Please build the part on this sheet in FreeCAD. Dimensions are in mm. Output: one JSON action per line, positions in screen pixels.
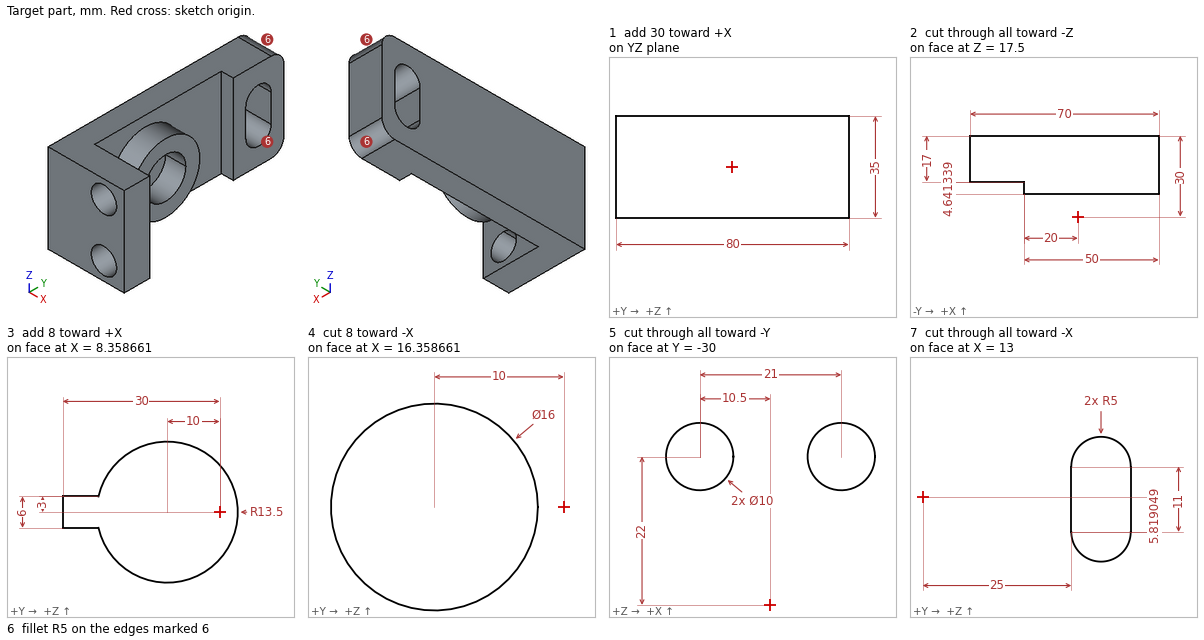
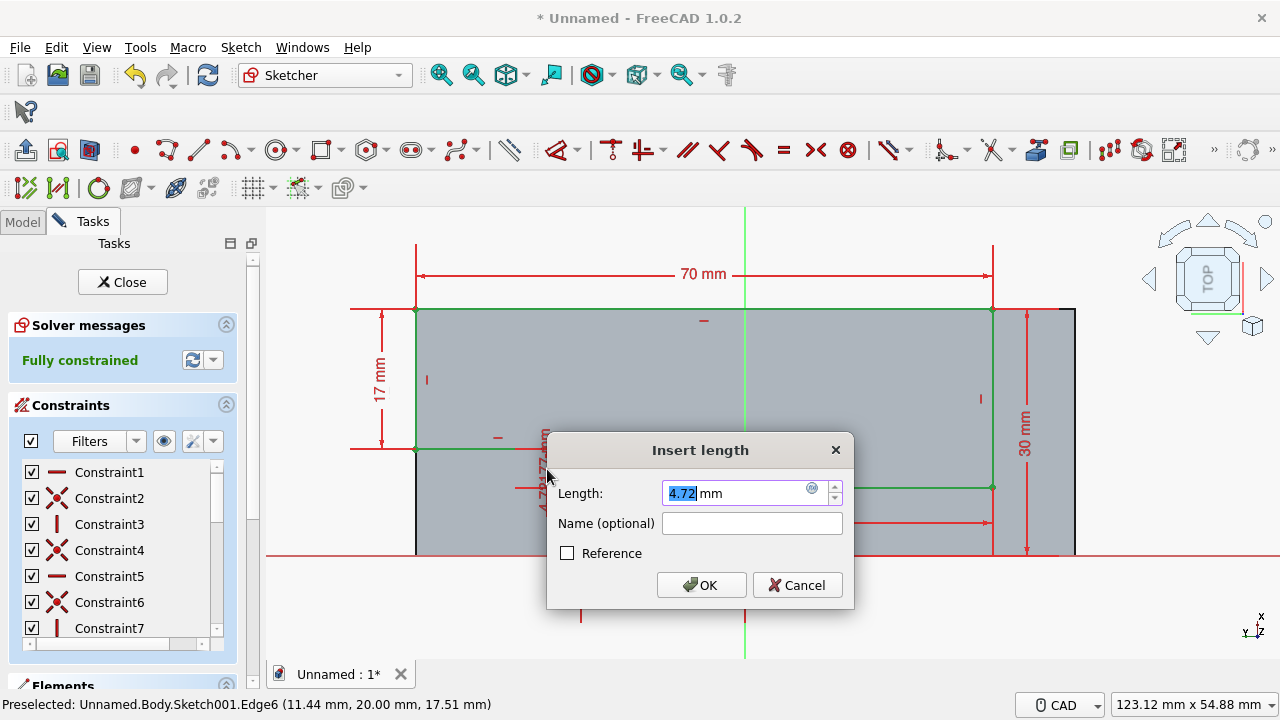
{"action": "type", "text": "4.641339"}
{"action": "key", "text": "Return"}
{"action": "key", "text": "Escape"}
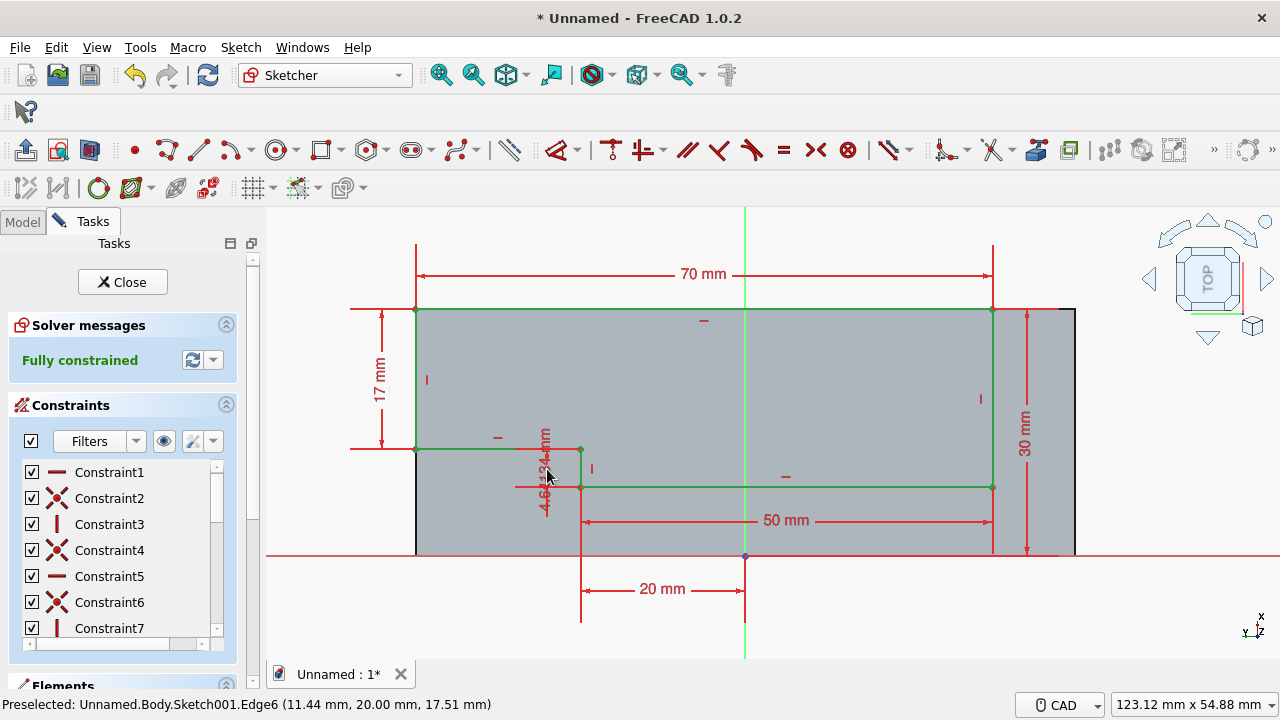
{"action": "left_click", "coordinate": [123, 282]}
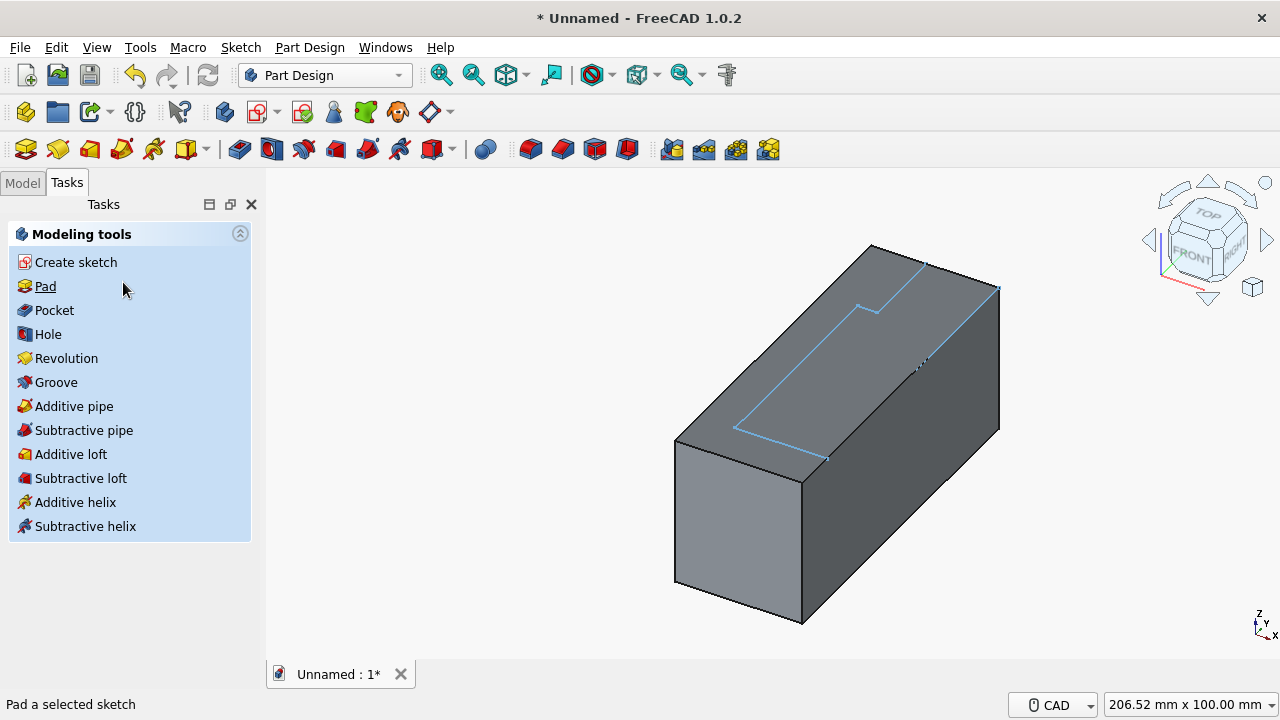
{"action": "left_click", "coordinate": [240, 150]}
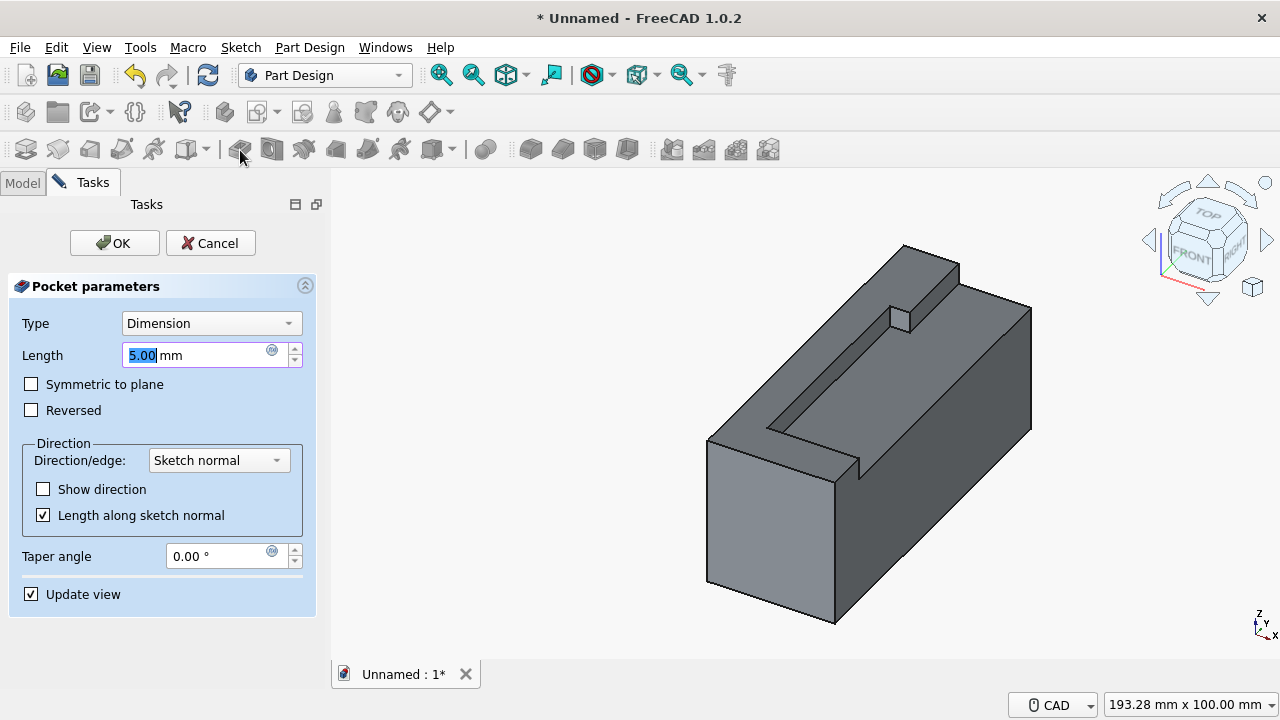
{"action": "left_click", "coordinate": [212, 324]}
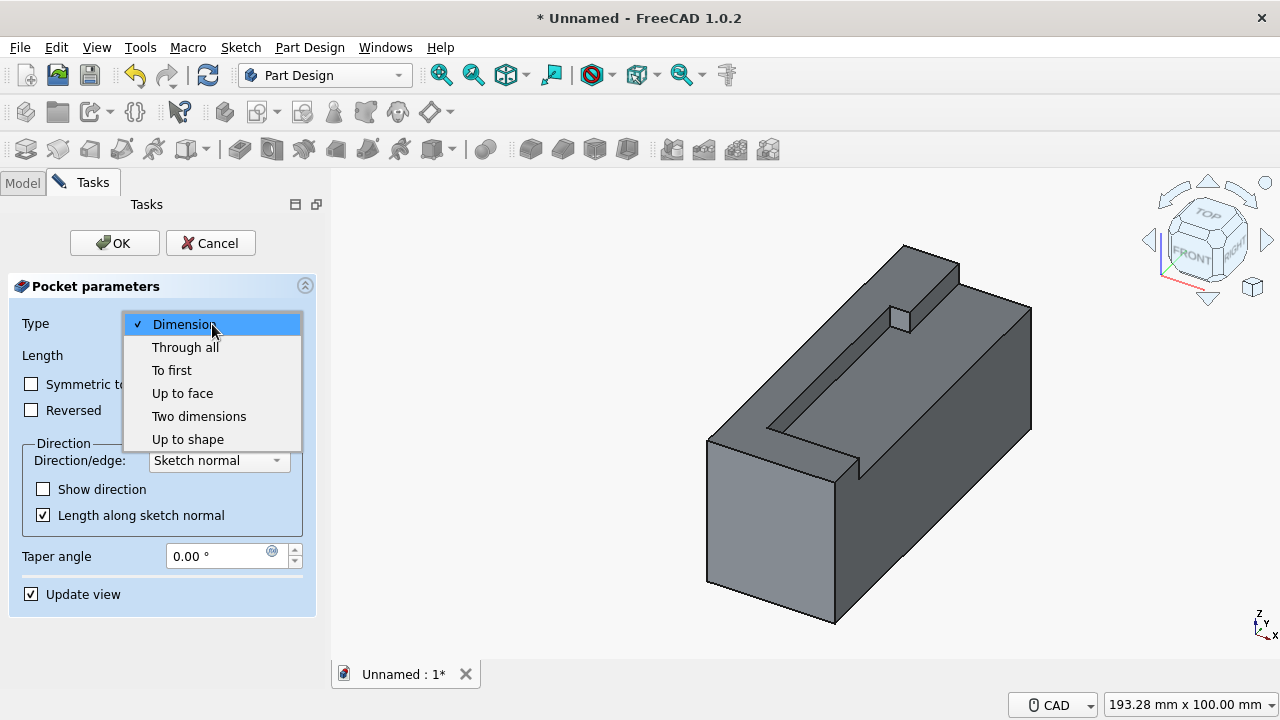
{"action": "left_click", "coordinate": [212, 348]}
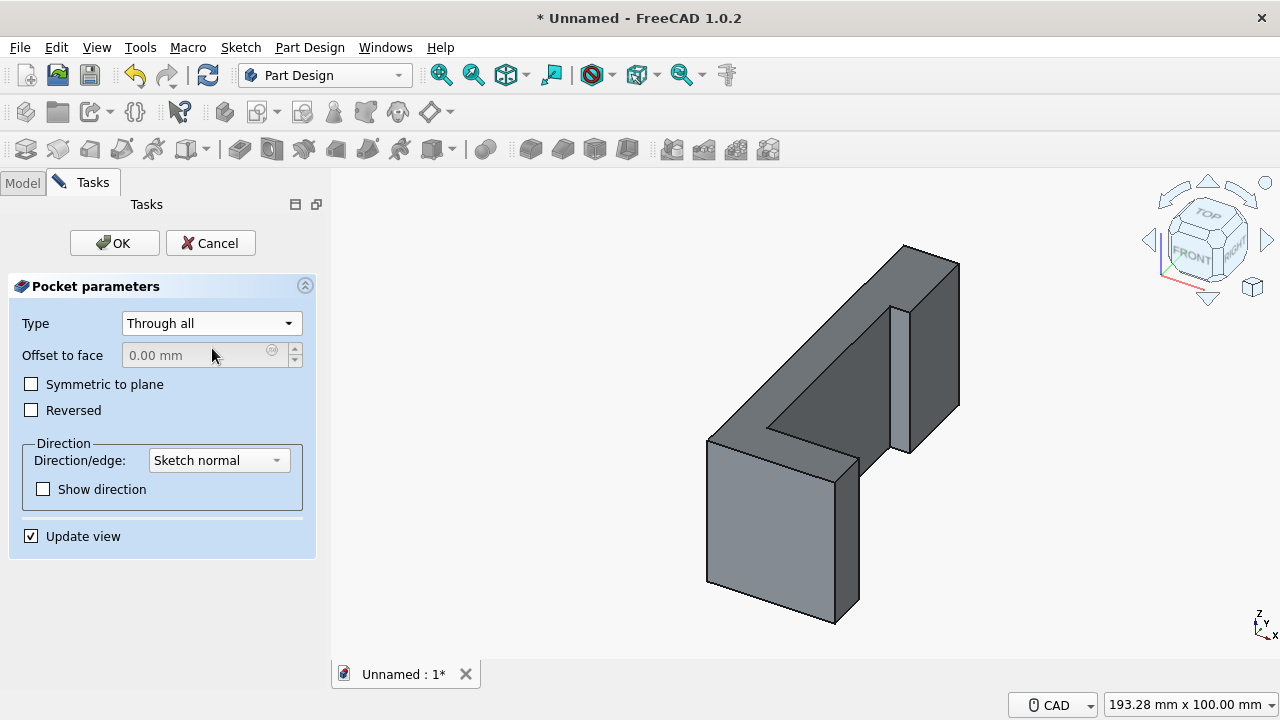
{"action": "left_click", "coordinate": [115, 243]}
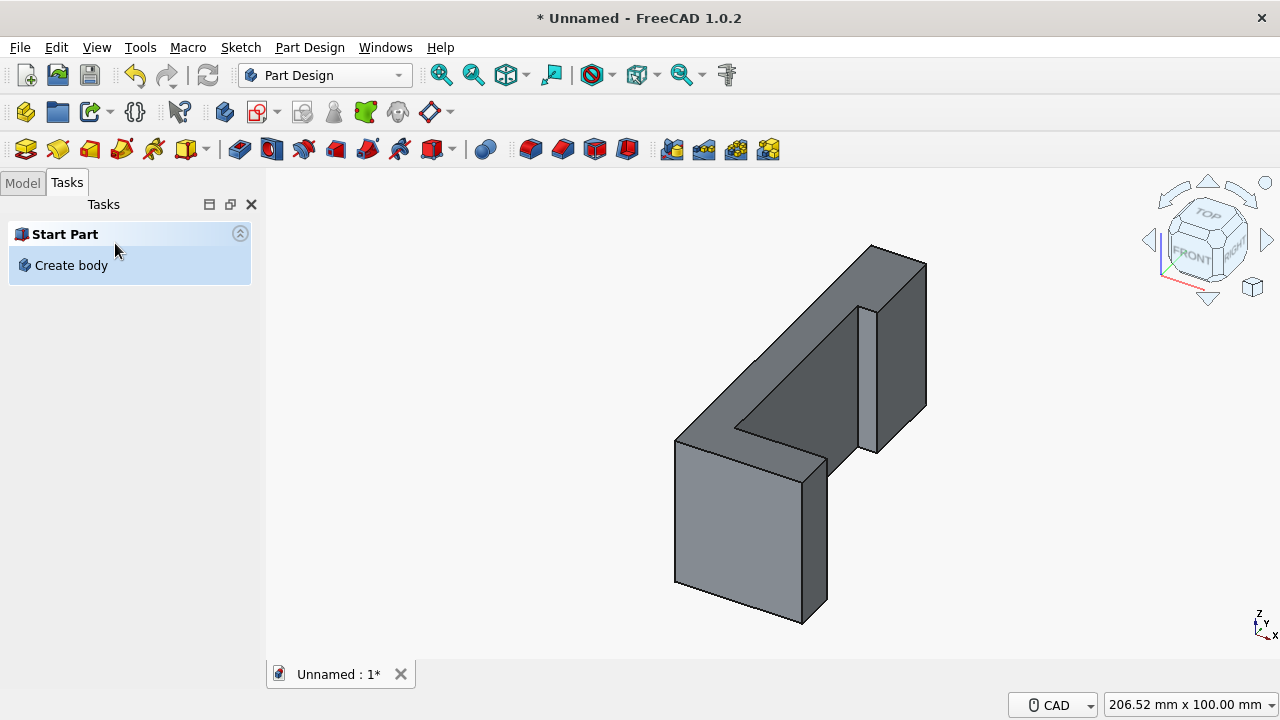
{"action": "left_click", "coordinate": [814, 419]}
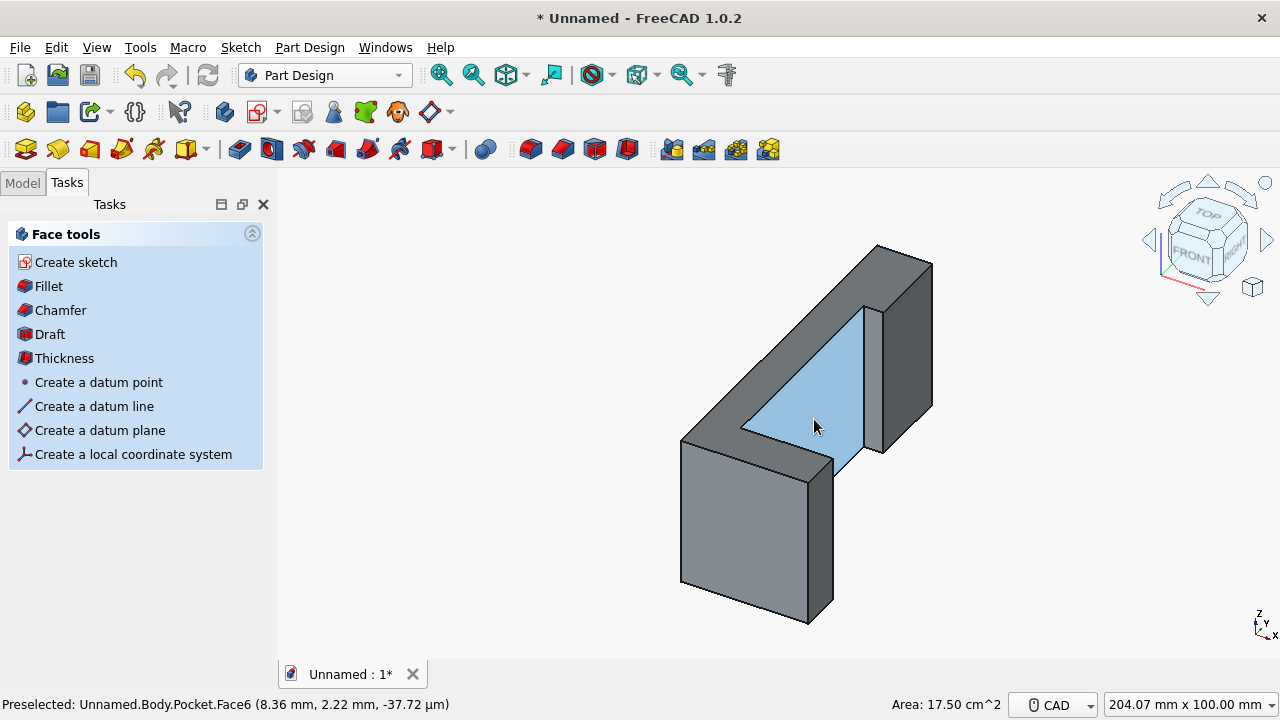
{"action": "left_click", "coordinate": [258, 112]}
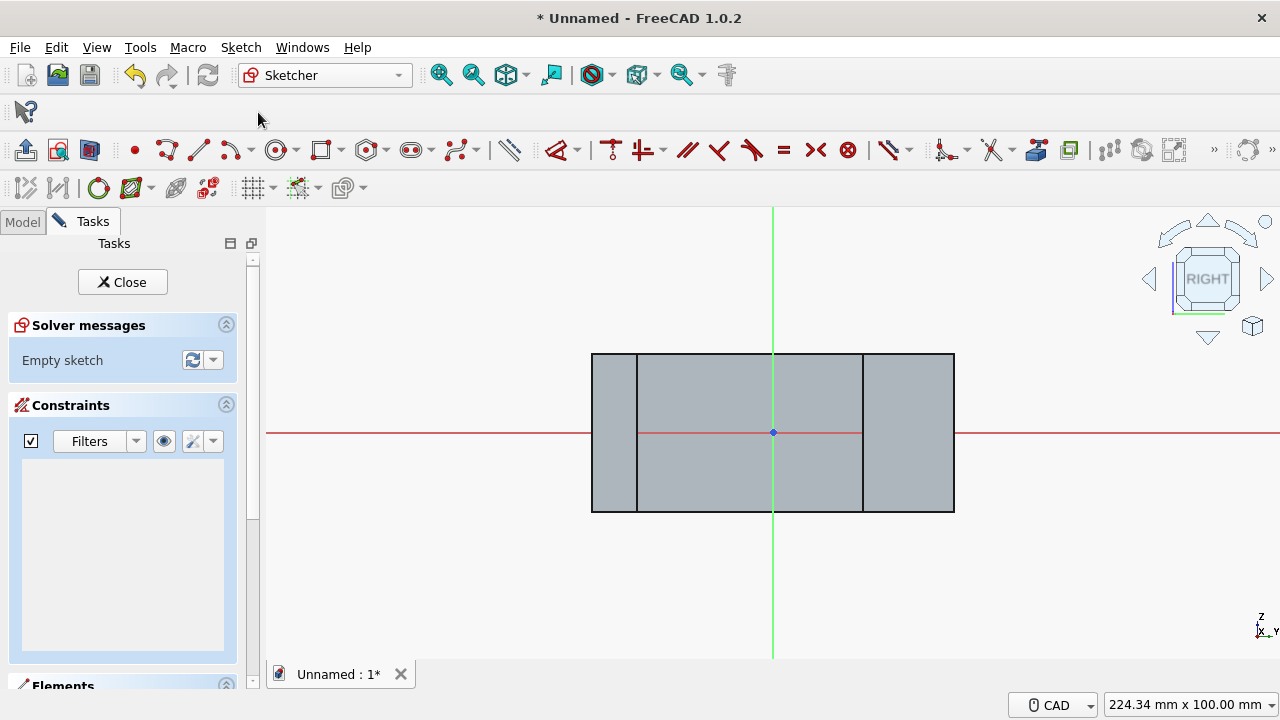
{"action": "scroll", "coordinate": [716, 433], "scroll_direction": "up", "scroll_amount": 7}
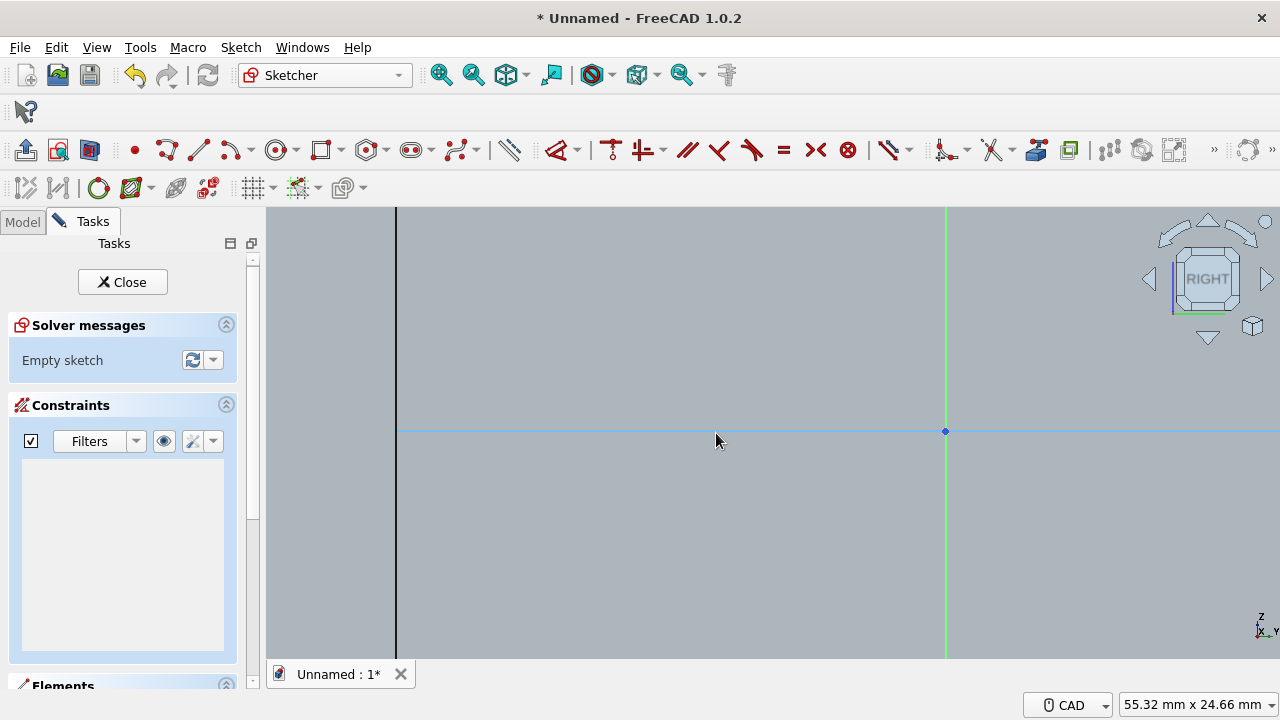
{"action": "left_click", "coordinate": [168, 150]}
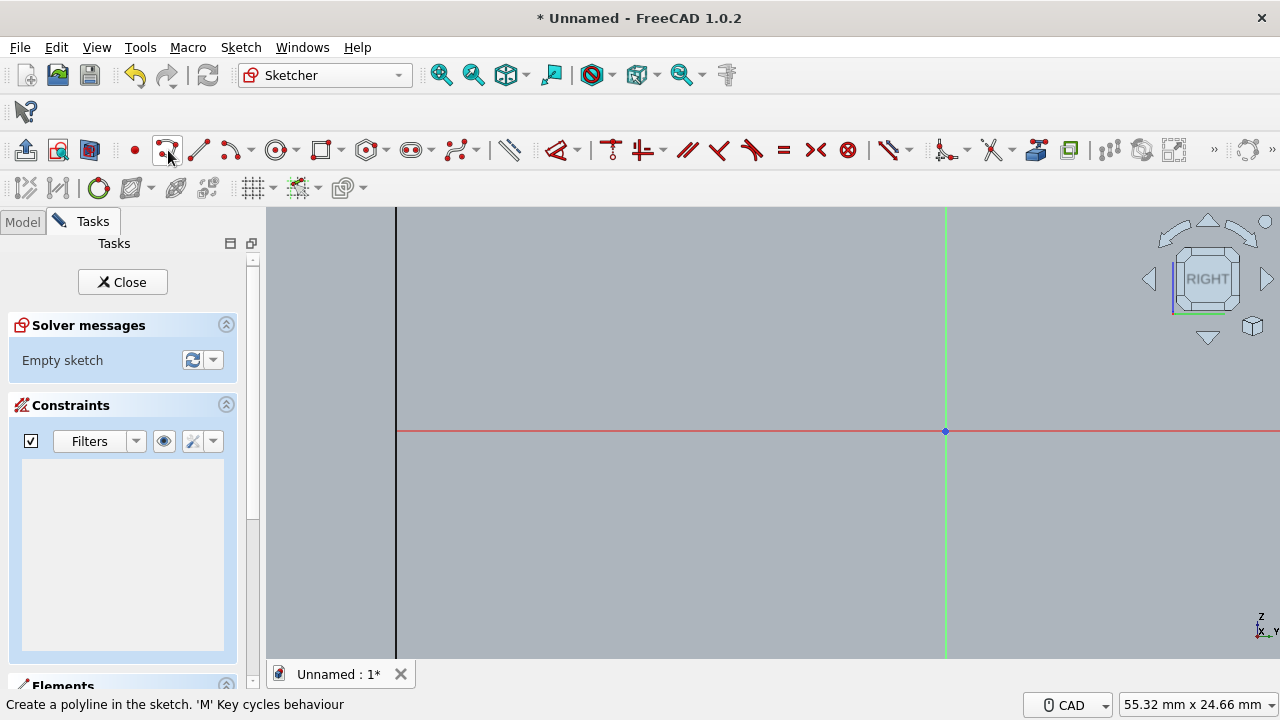
{"action": "left_click", "coordinate": [521, 376]}
{"action": "left_click", "coordinate": [396, 376]}
{"action": "left_click", "coordinate": [396, 486]}
{"action": "left_click", "coordinate": [521, 486]}
{"action": "right_click", "coordinate": [521, 486]}